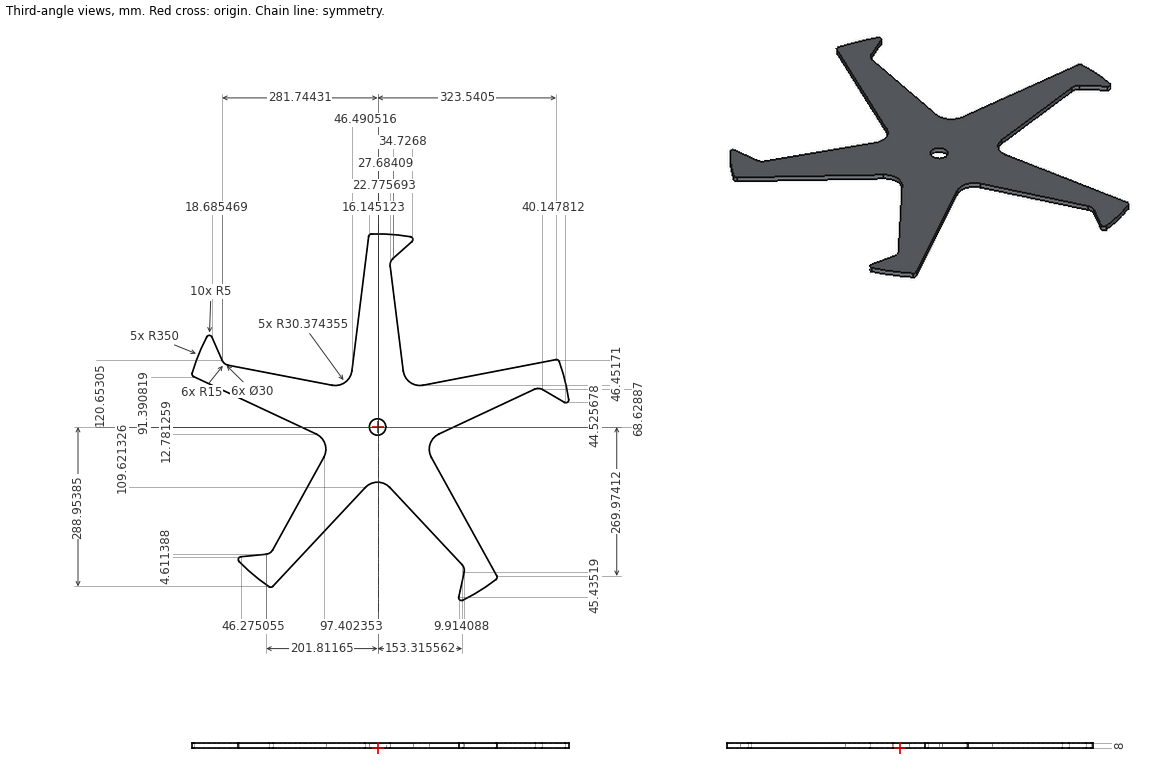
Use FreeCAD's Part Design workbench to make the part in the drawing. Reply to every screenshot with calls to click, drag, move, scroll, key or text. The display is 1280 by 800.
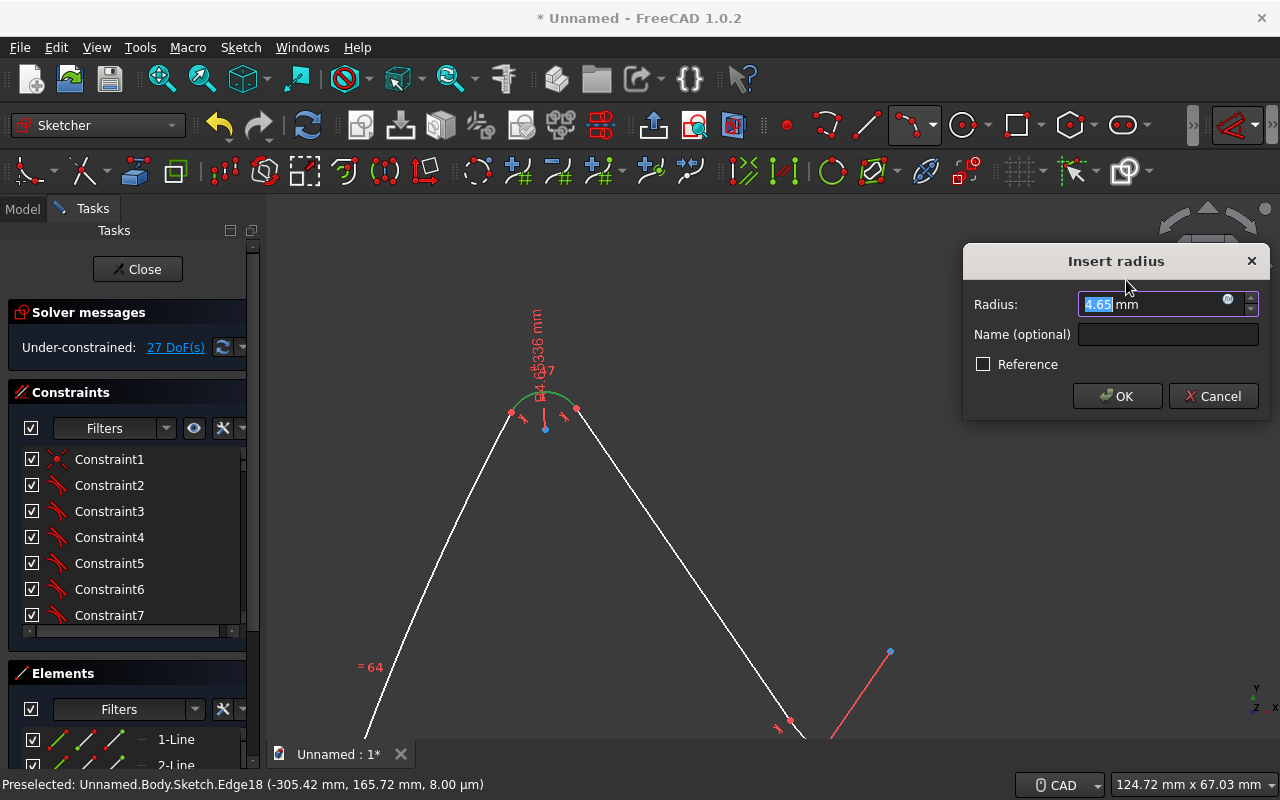
text(5)
key(Return)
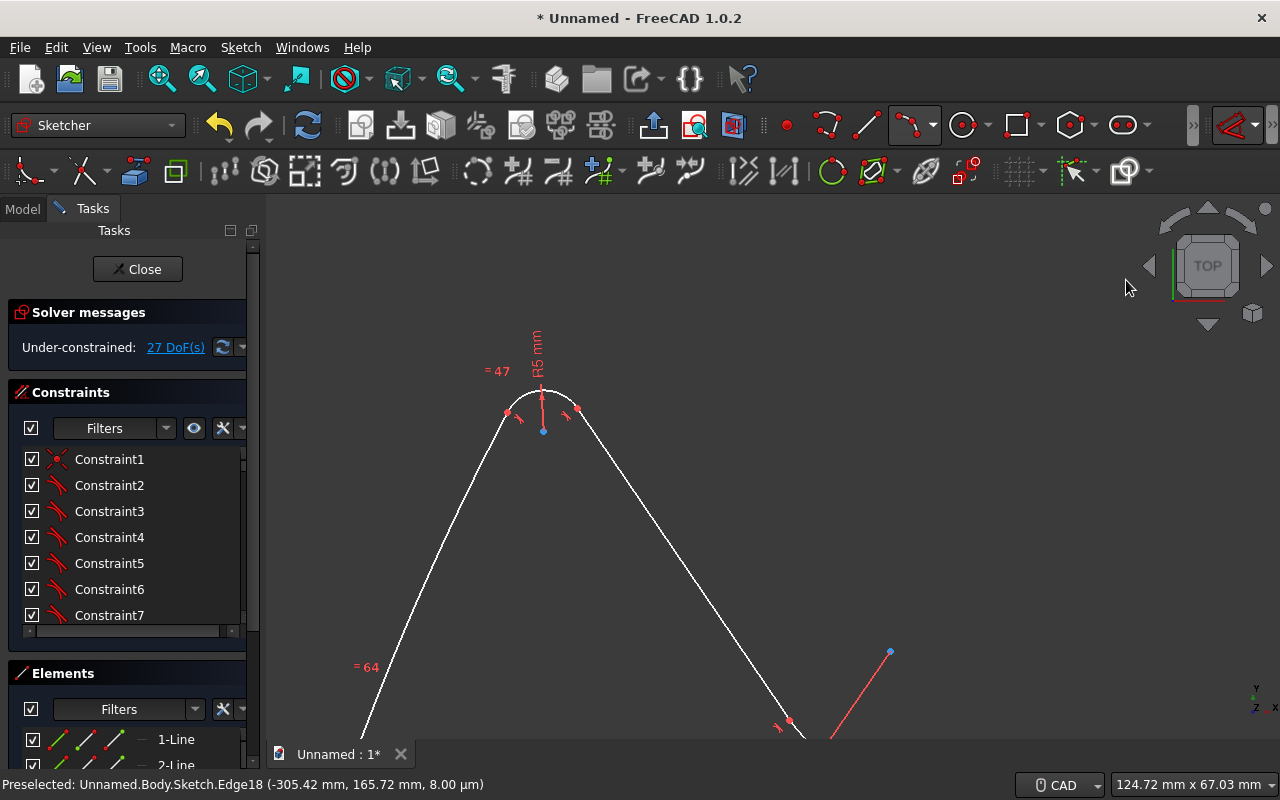
scroll(551, 393, down, 14)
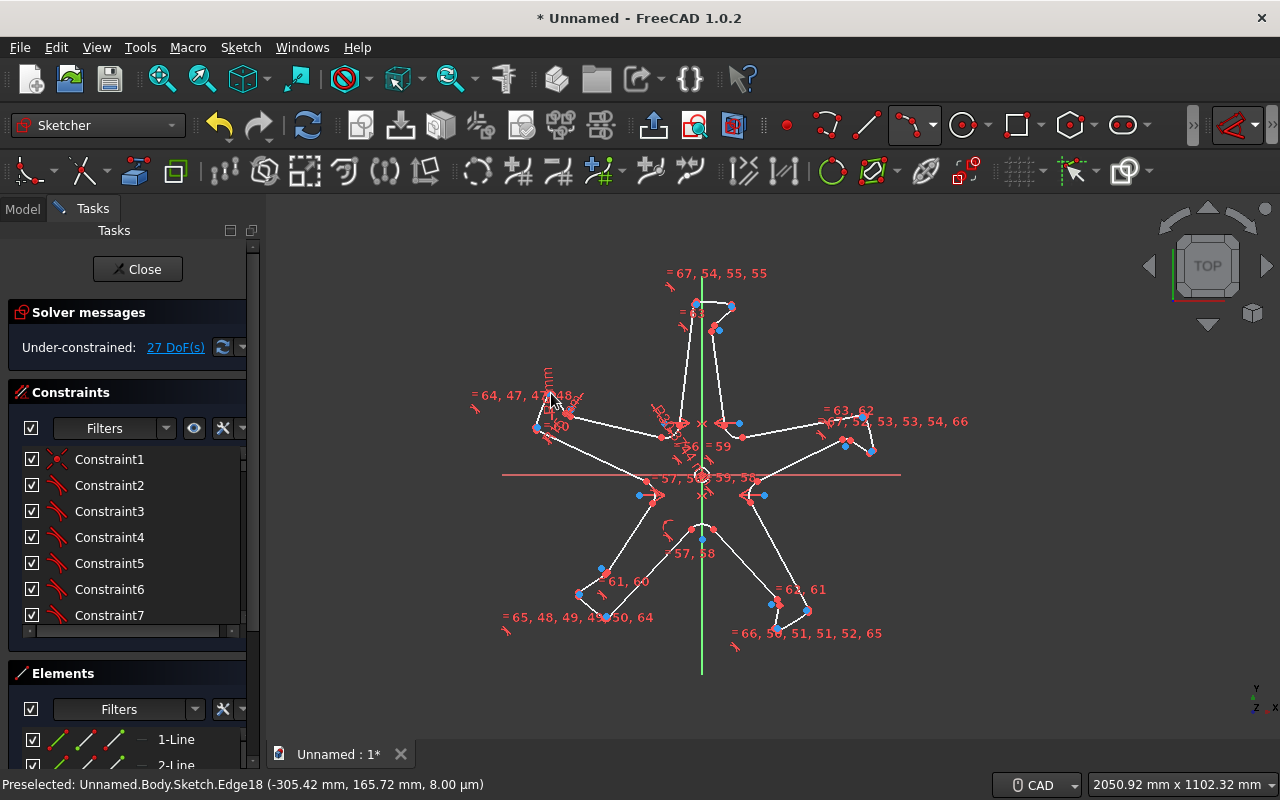
scroll(544, 404, up, 2)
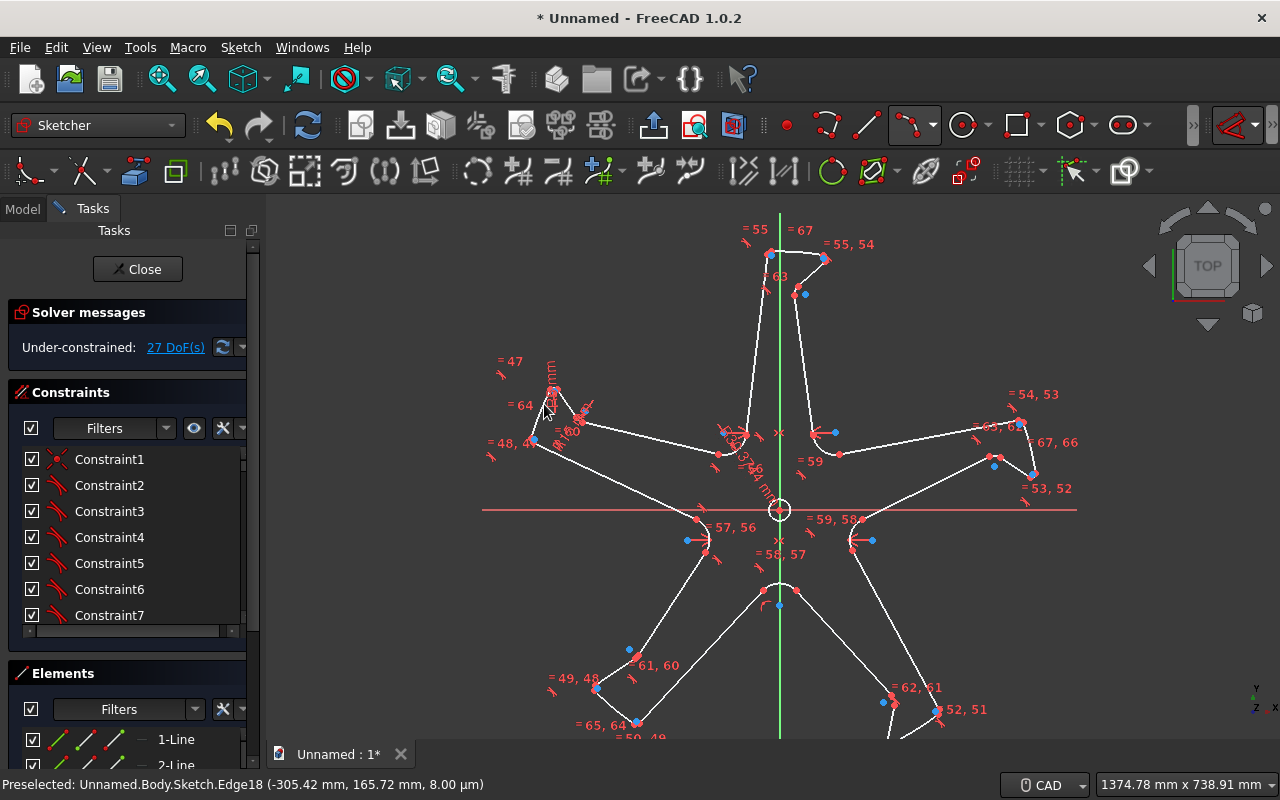
click(544, 404)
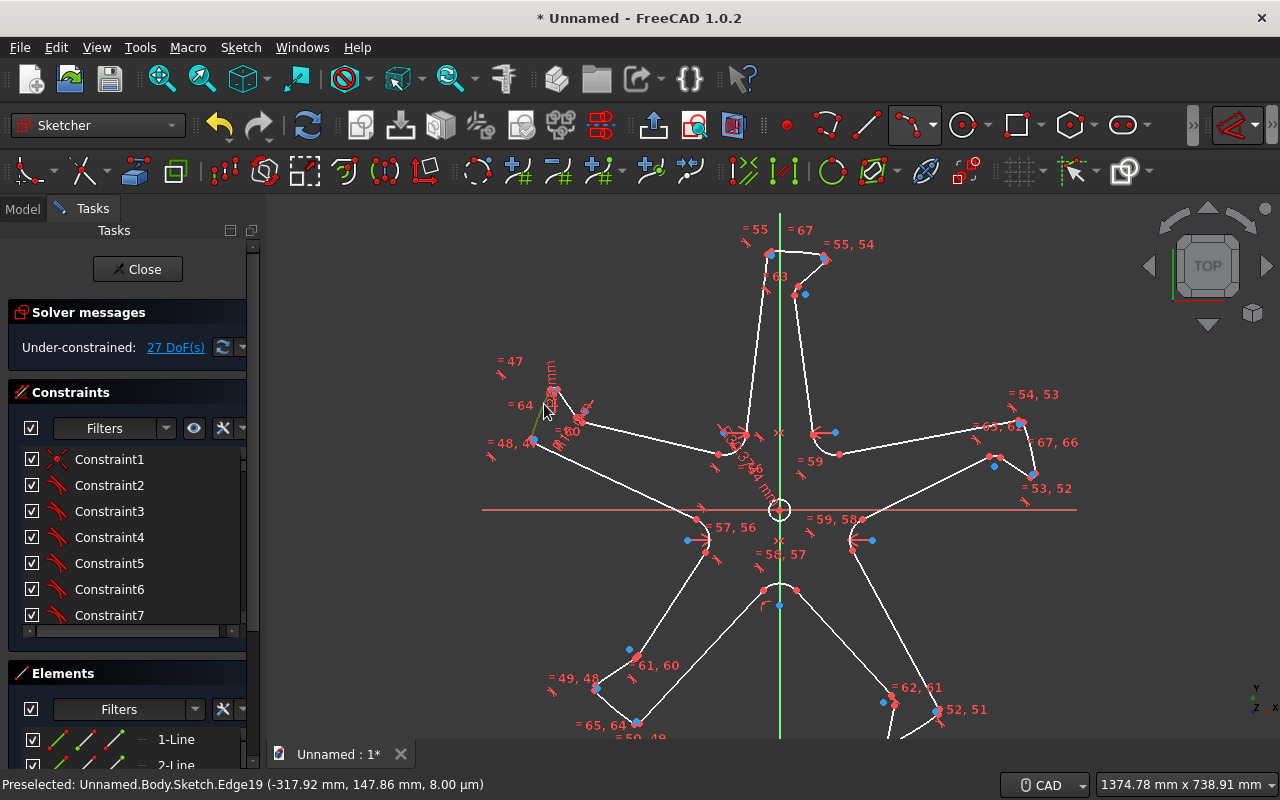
click(1258, 126)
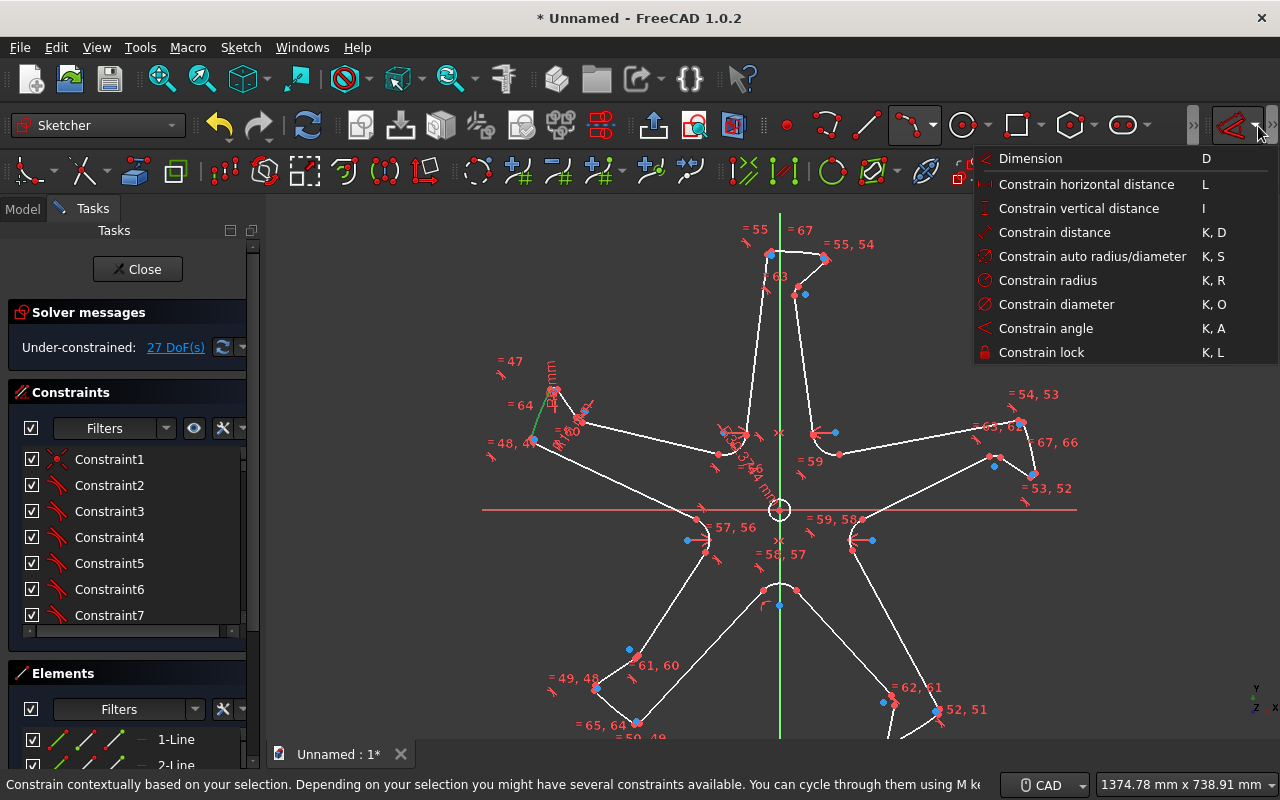
click(1126, 280)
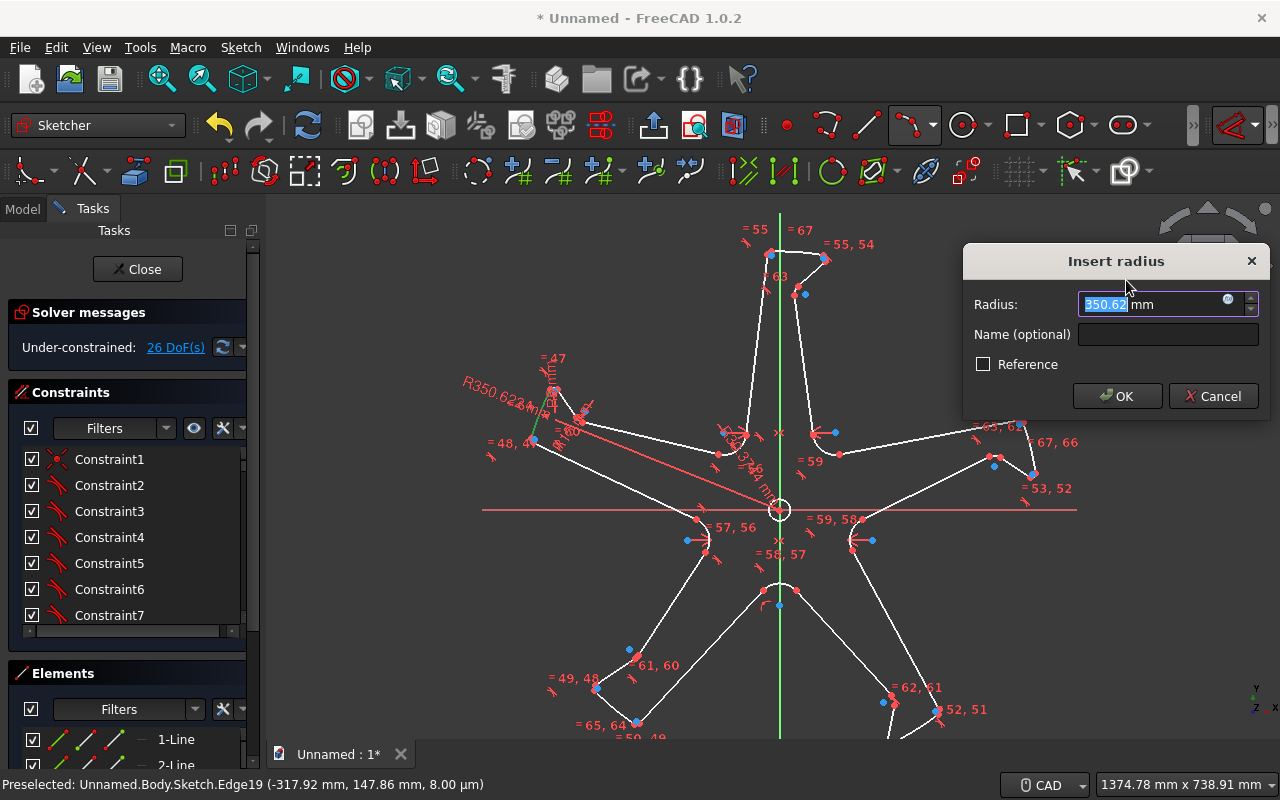
text(350)
key(Return)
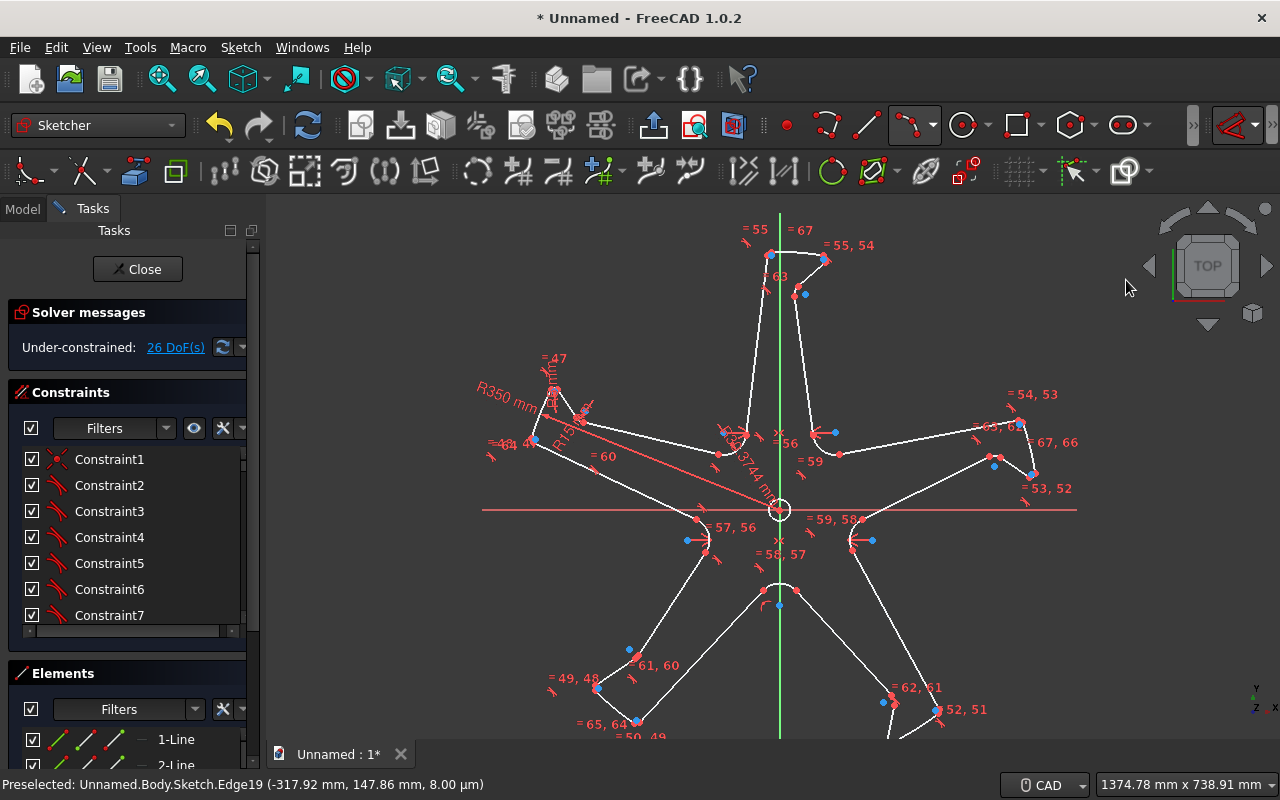
scroll(780, 499, up, 3)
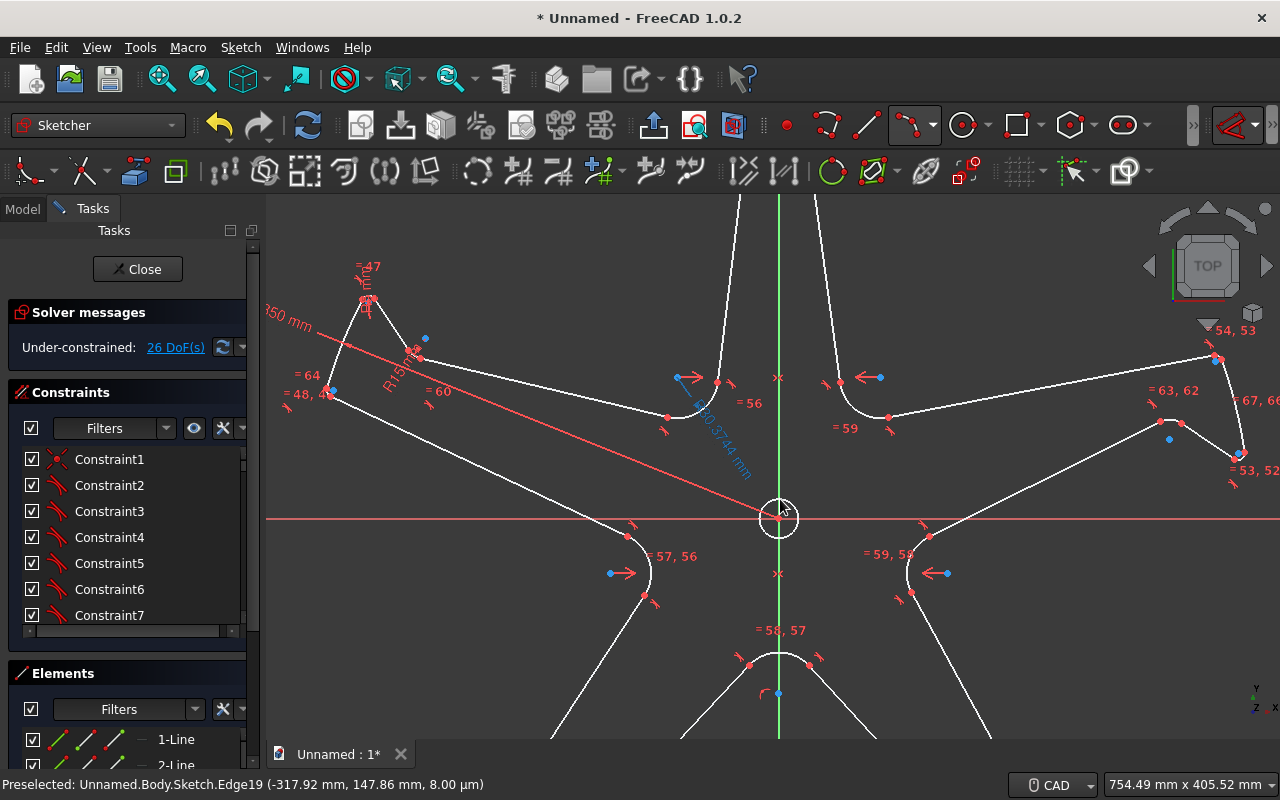
click(780, 499)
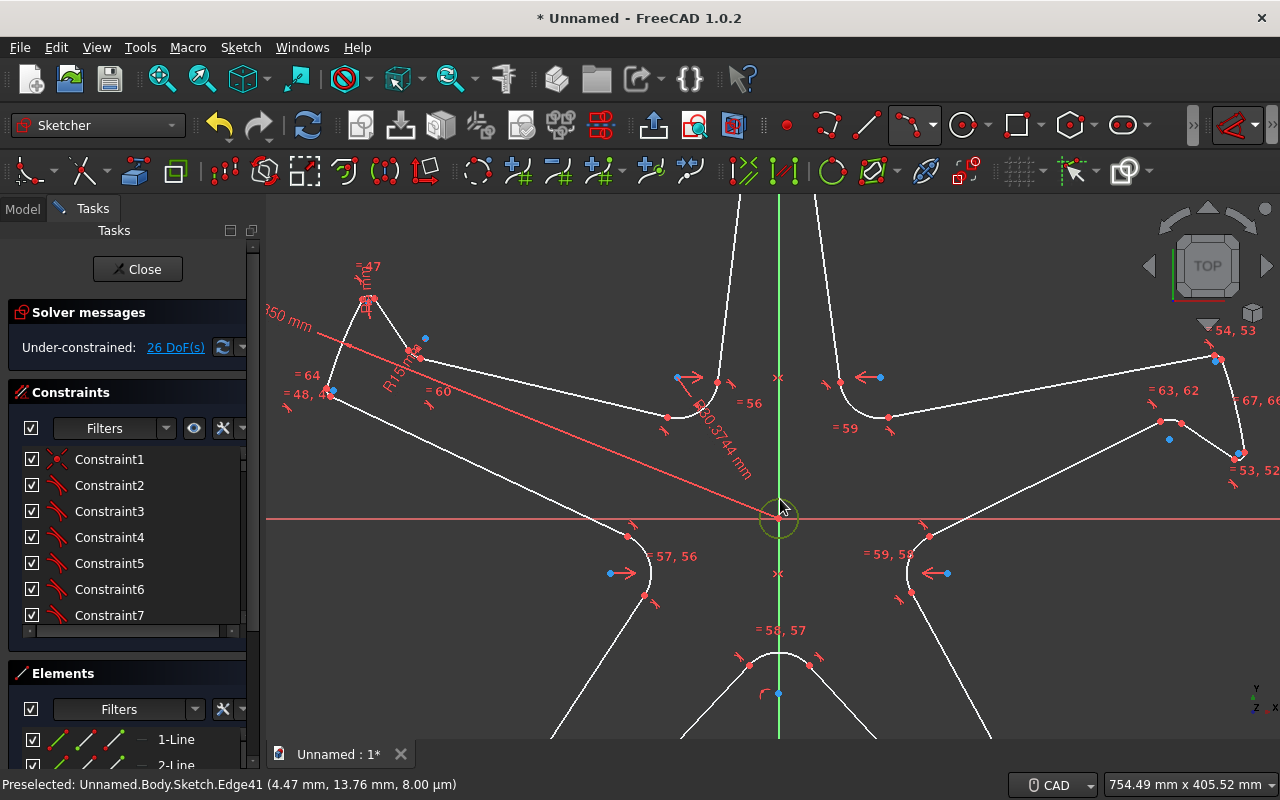
click(1258, 126)